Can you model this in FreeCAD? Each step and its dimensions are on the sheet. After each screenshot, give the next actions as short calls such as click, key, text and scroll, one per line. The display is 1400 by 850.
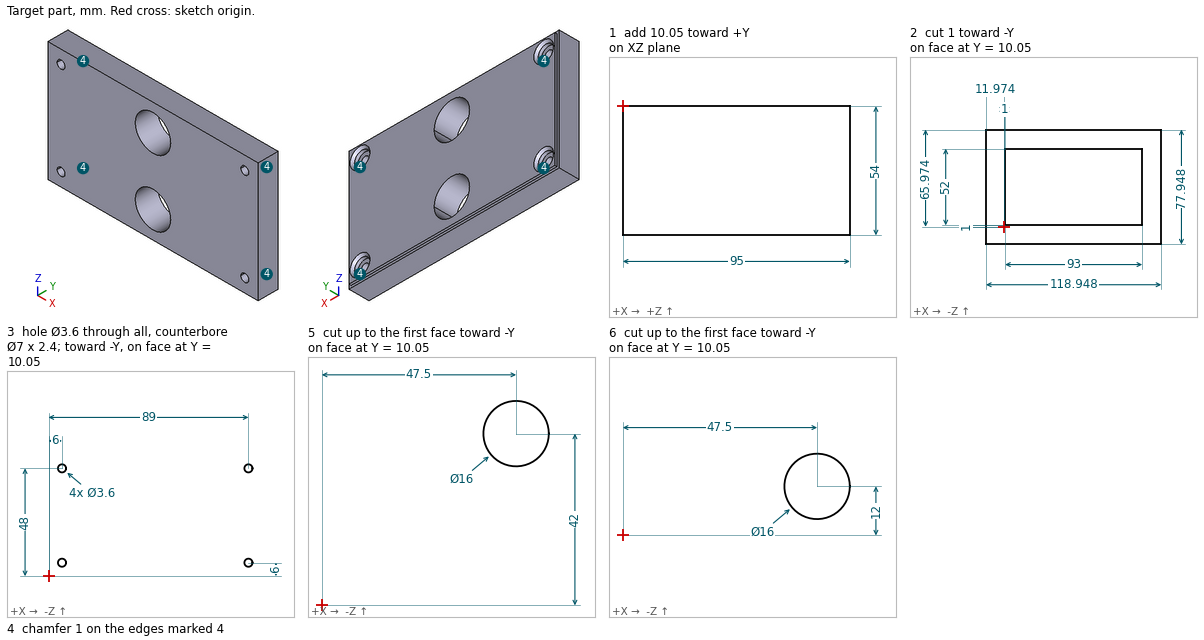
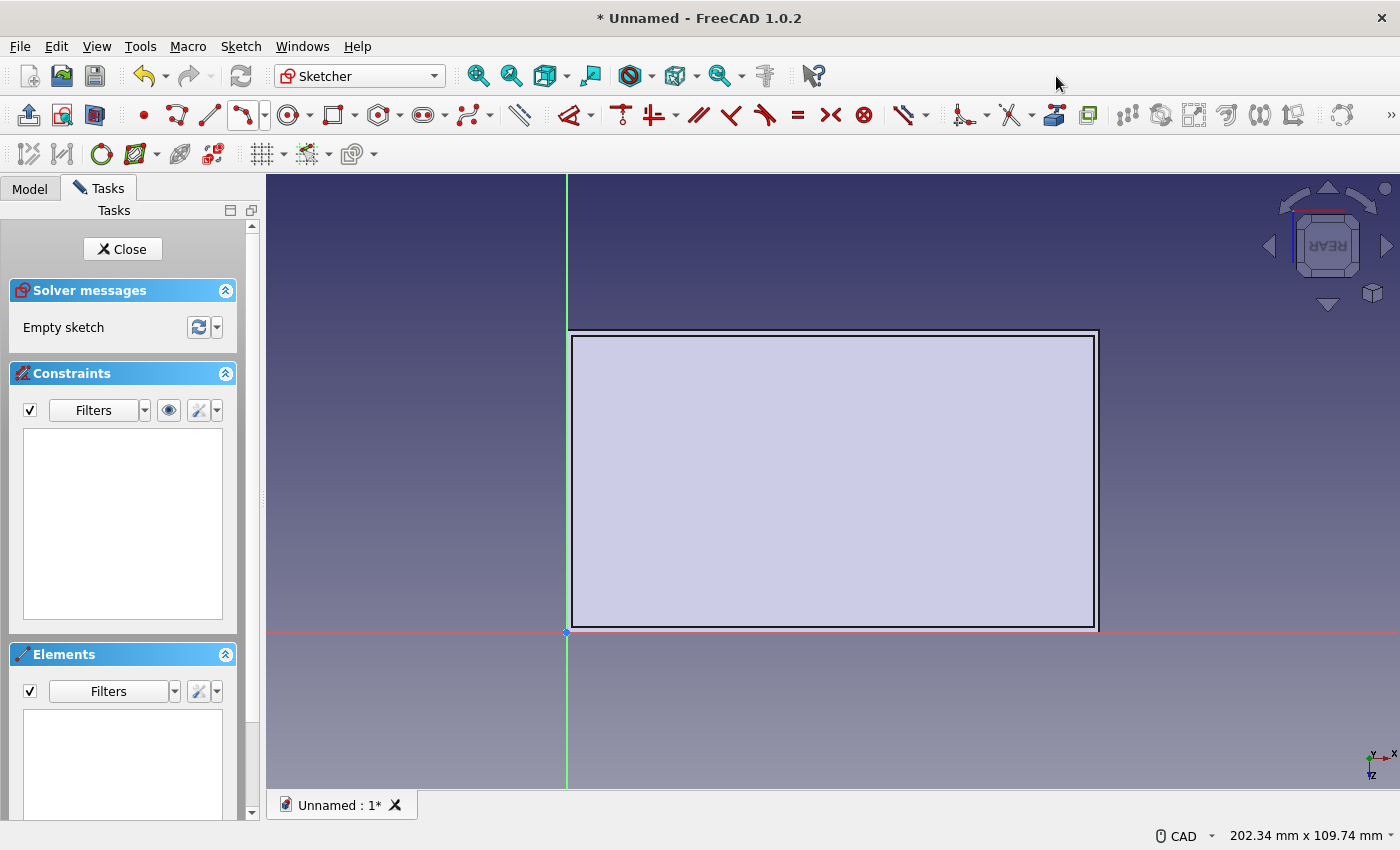
click(288, 116)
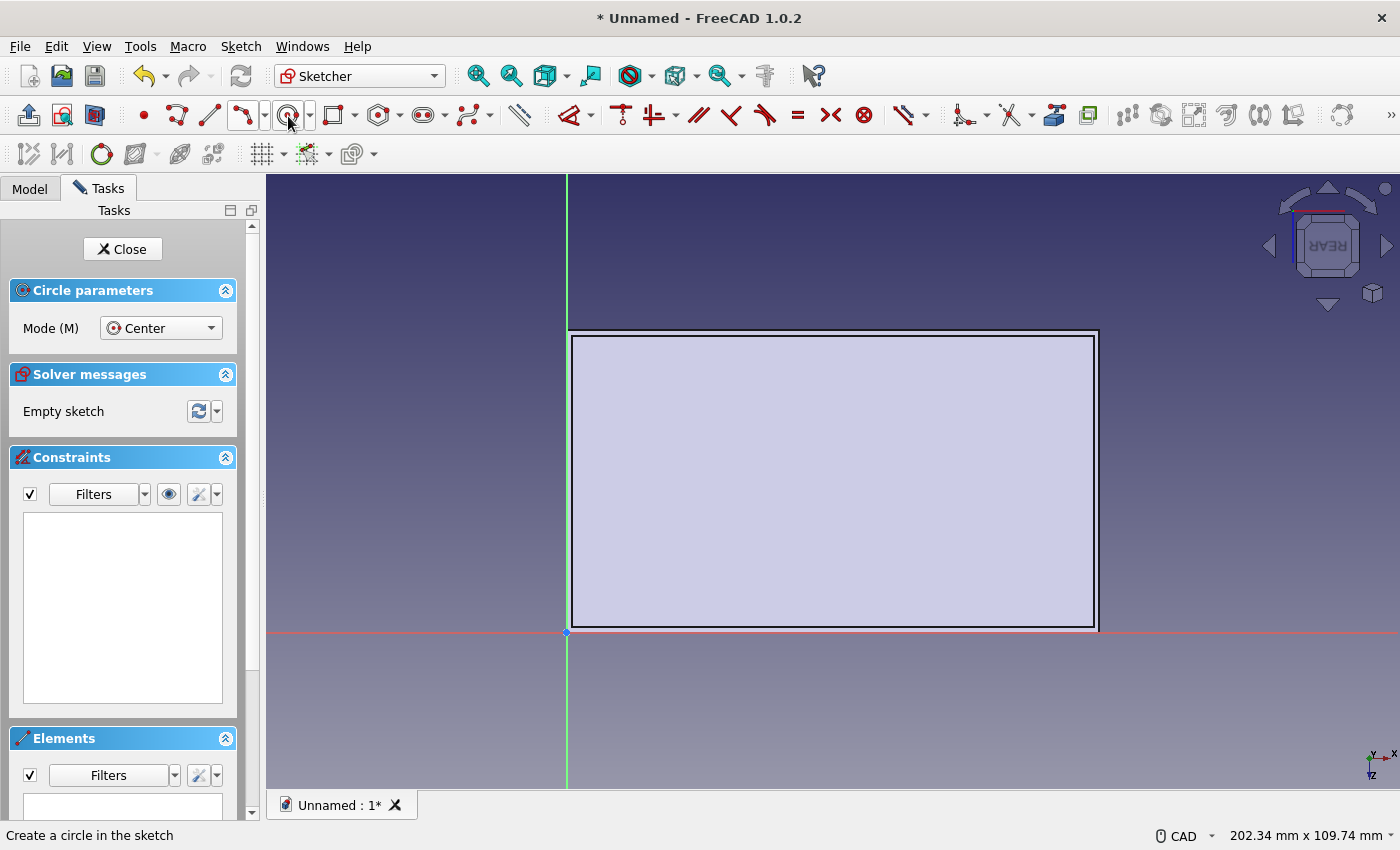
scroll(600, 364, up, 5)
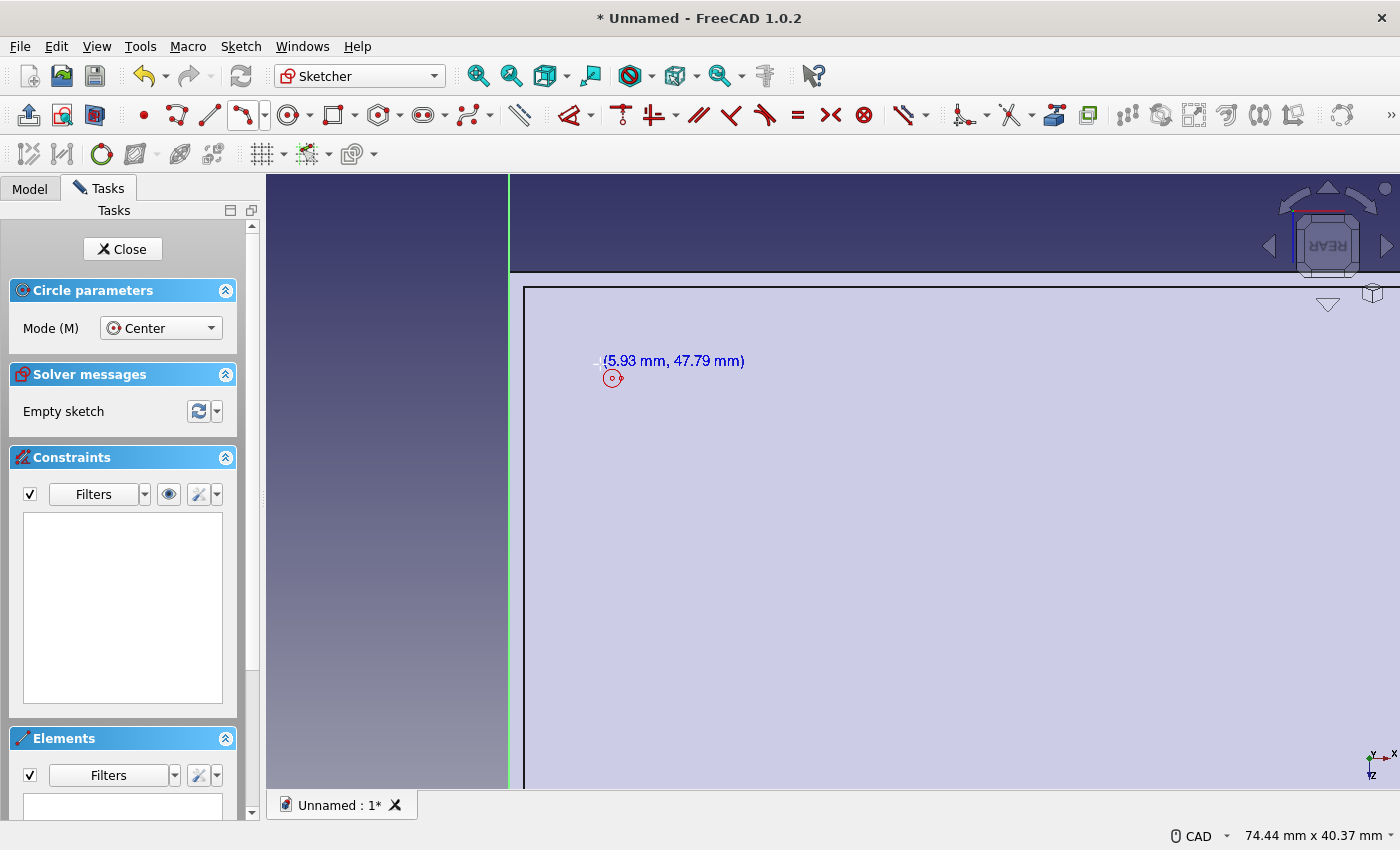
click(601, 363)
move(620, 344)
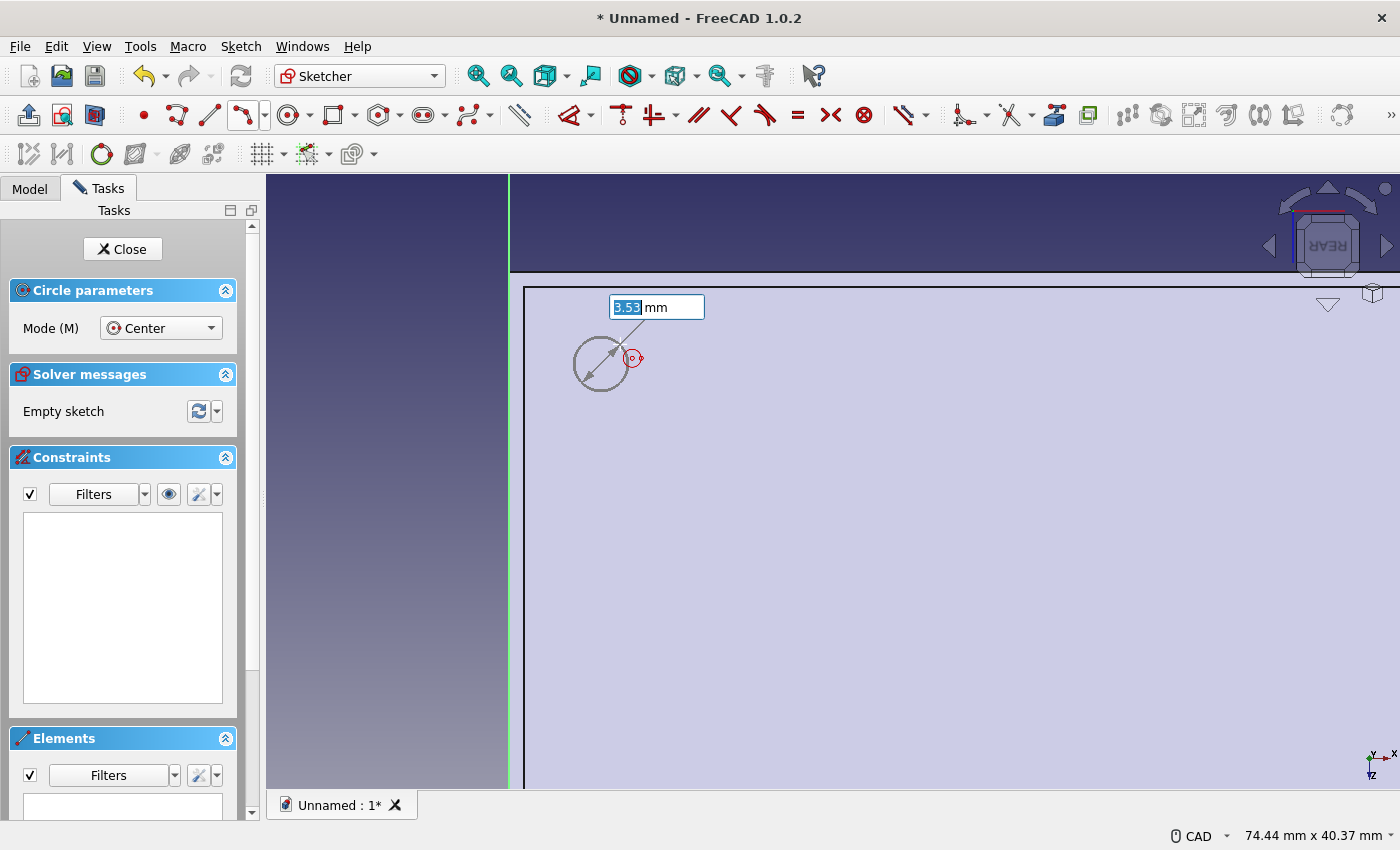
text(3.6)
key(Return)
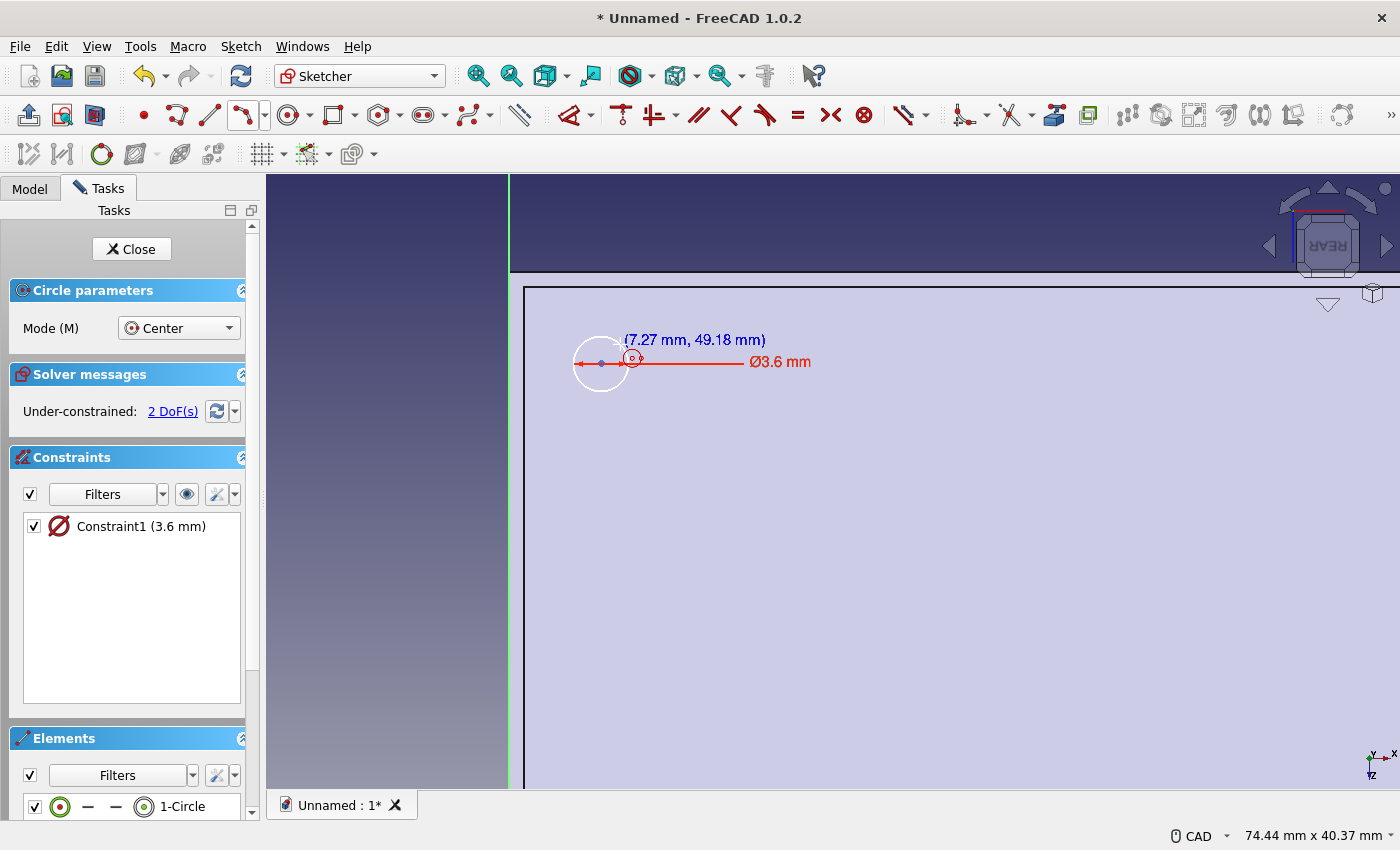
scroll(408, 291, down, 4)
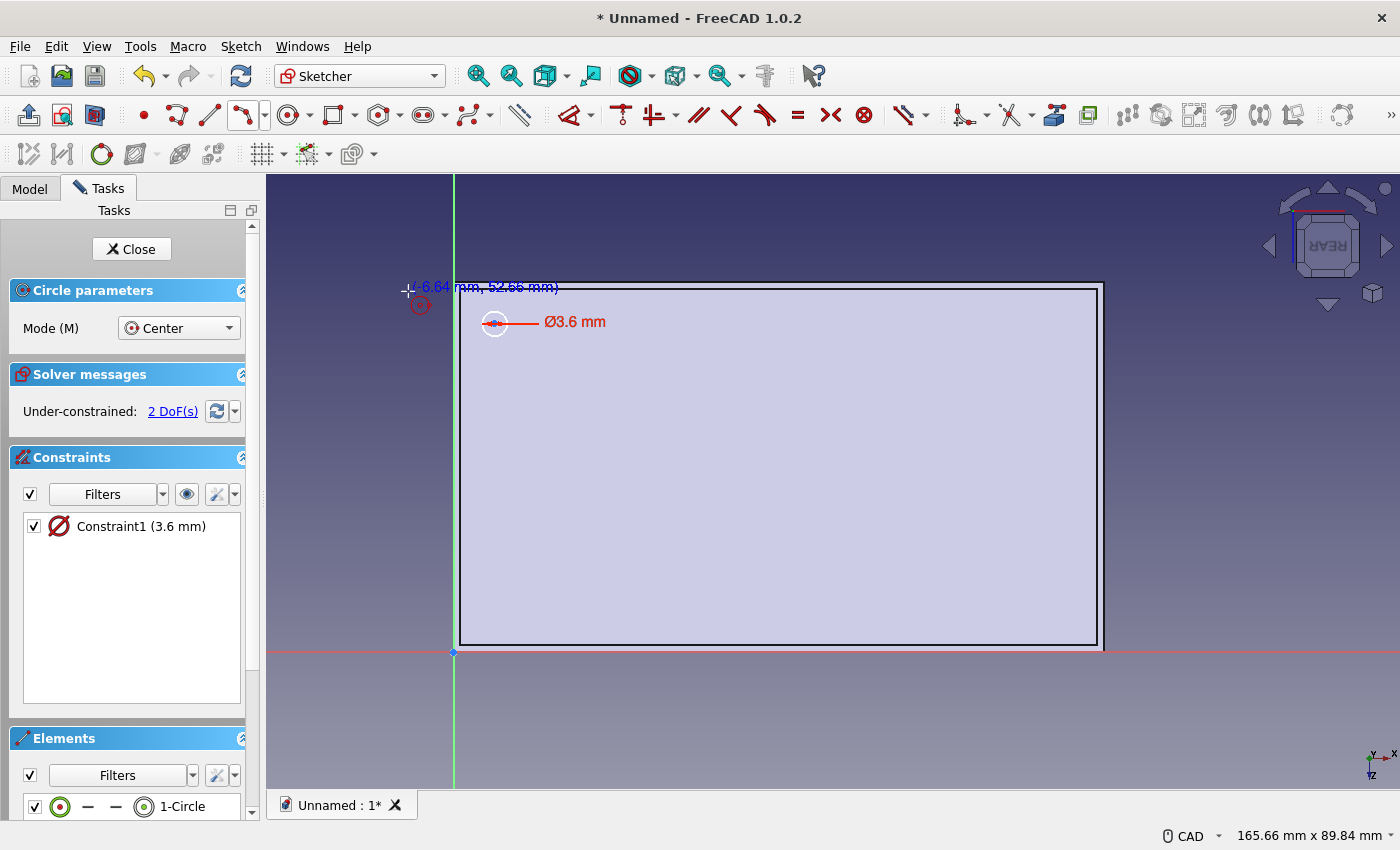
scroll(1063, 323, up, 4)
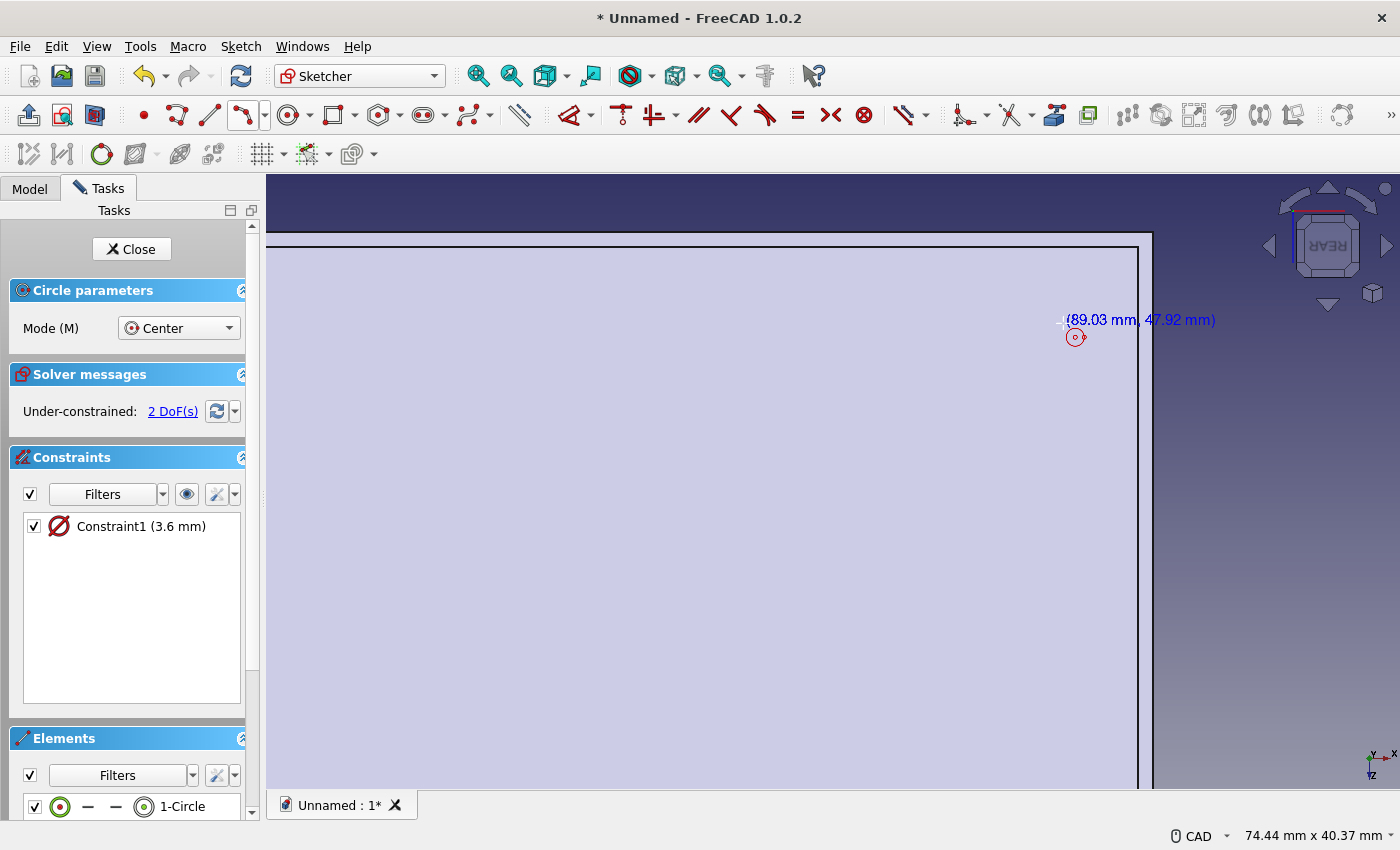
click(1062, 324)
move(1081, 304)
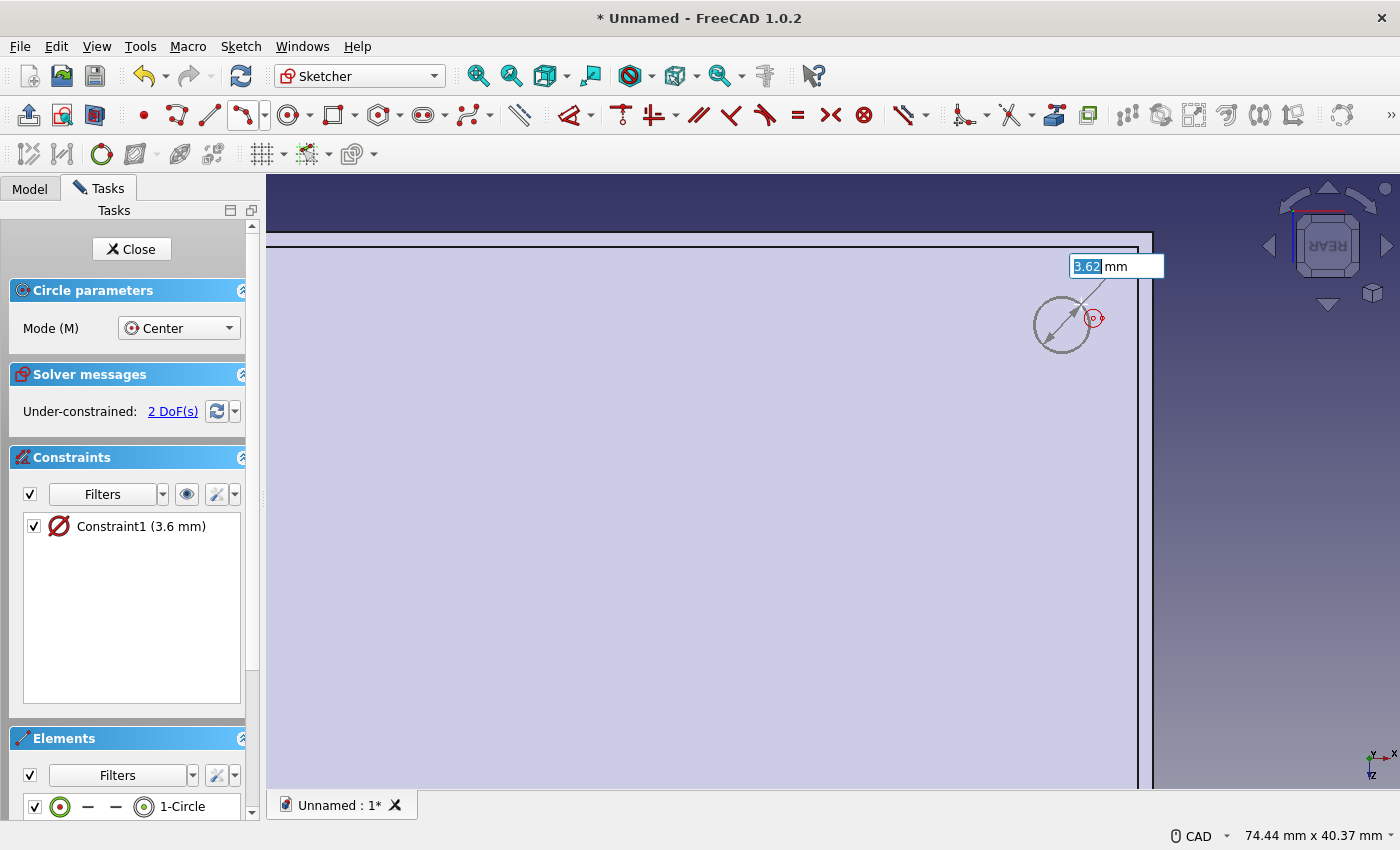
text(3.6)
key(Return)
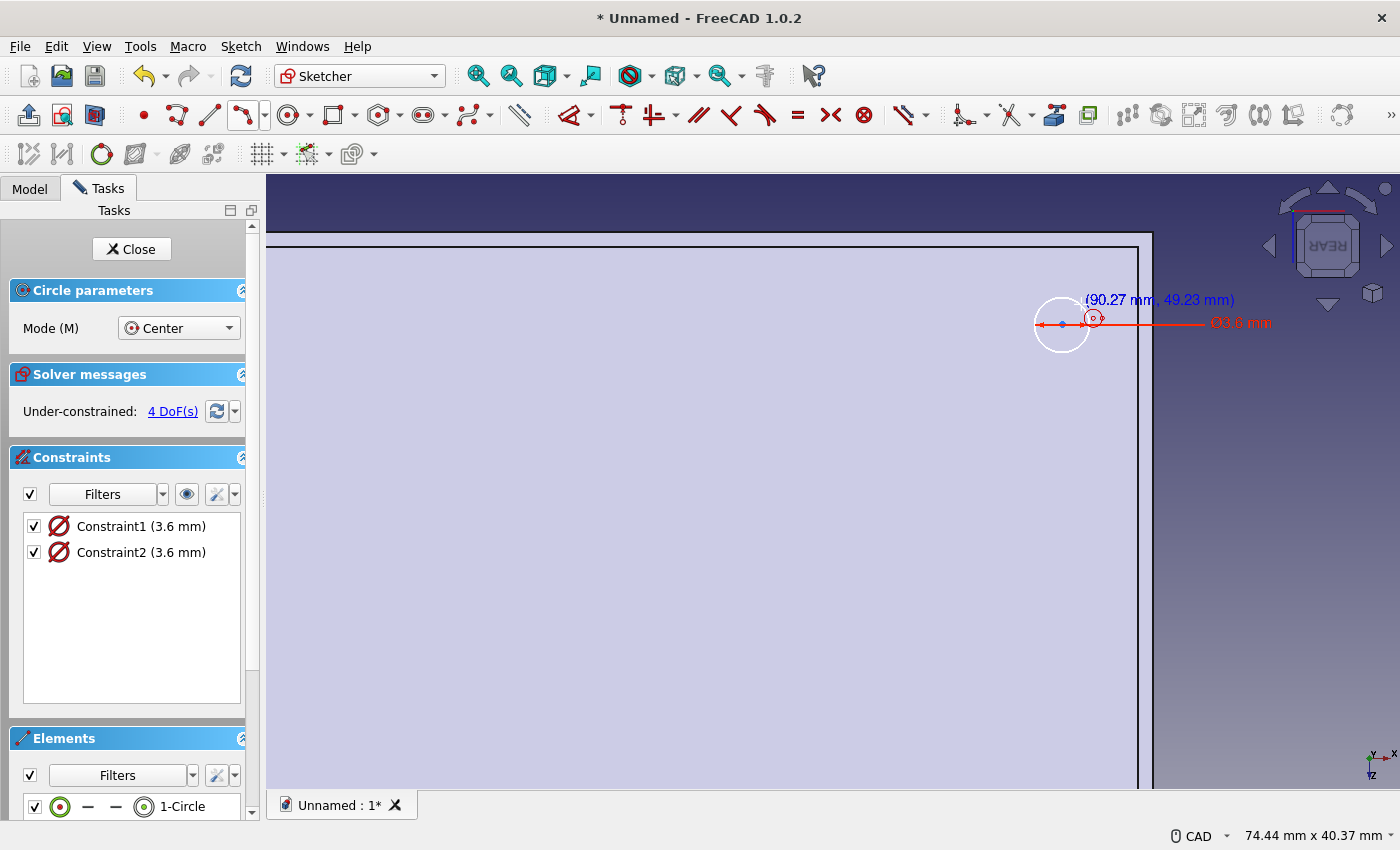
scroll(1064, 323, down, 4)